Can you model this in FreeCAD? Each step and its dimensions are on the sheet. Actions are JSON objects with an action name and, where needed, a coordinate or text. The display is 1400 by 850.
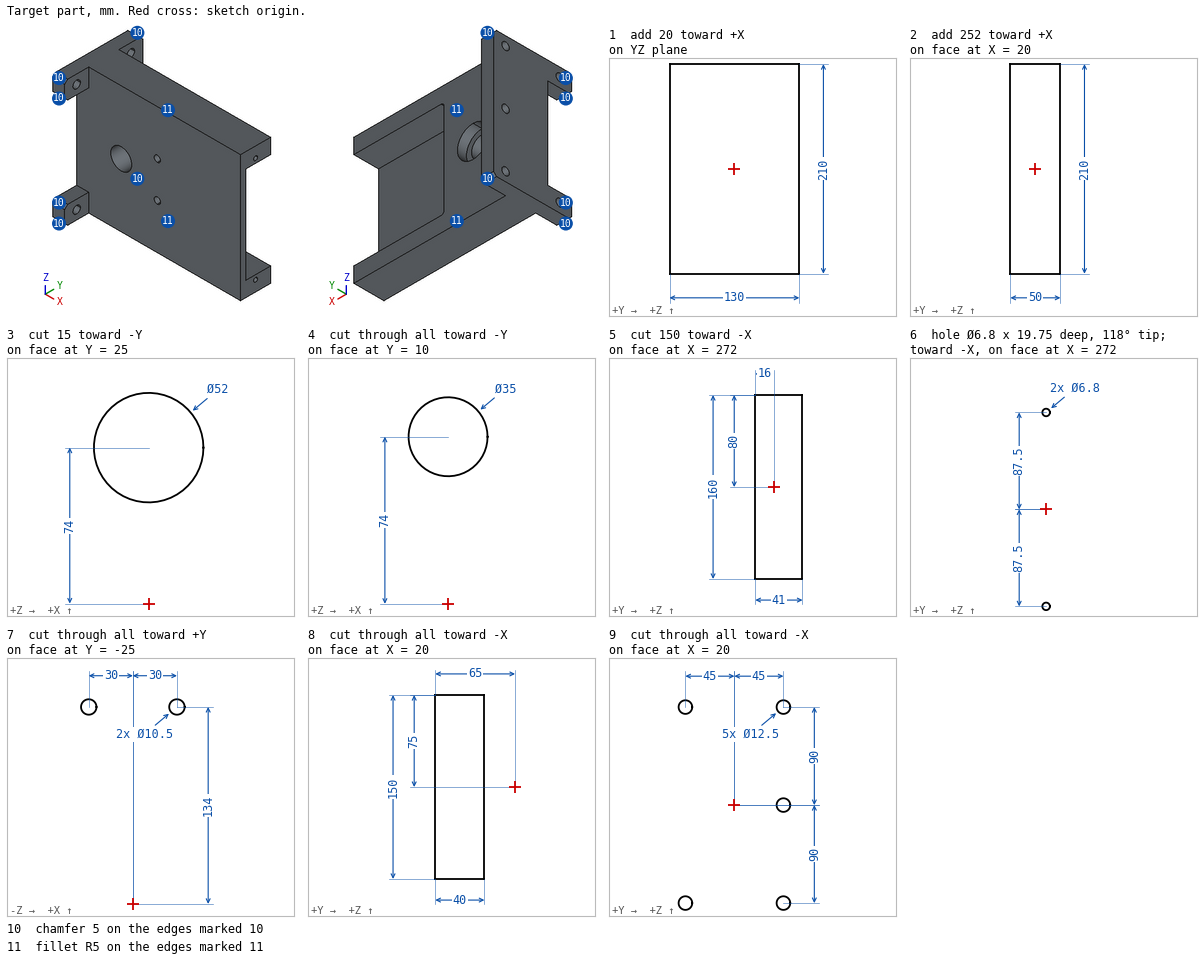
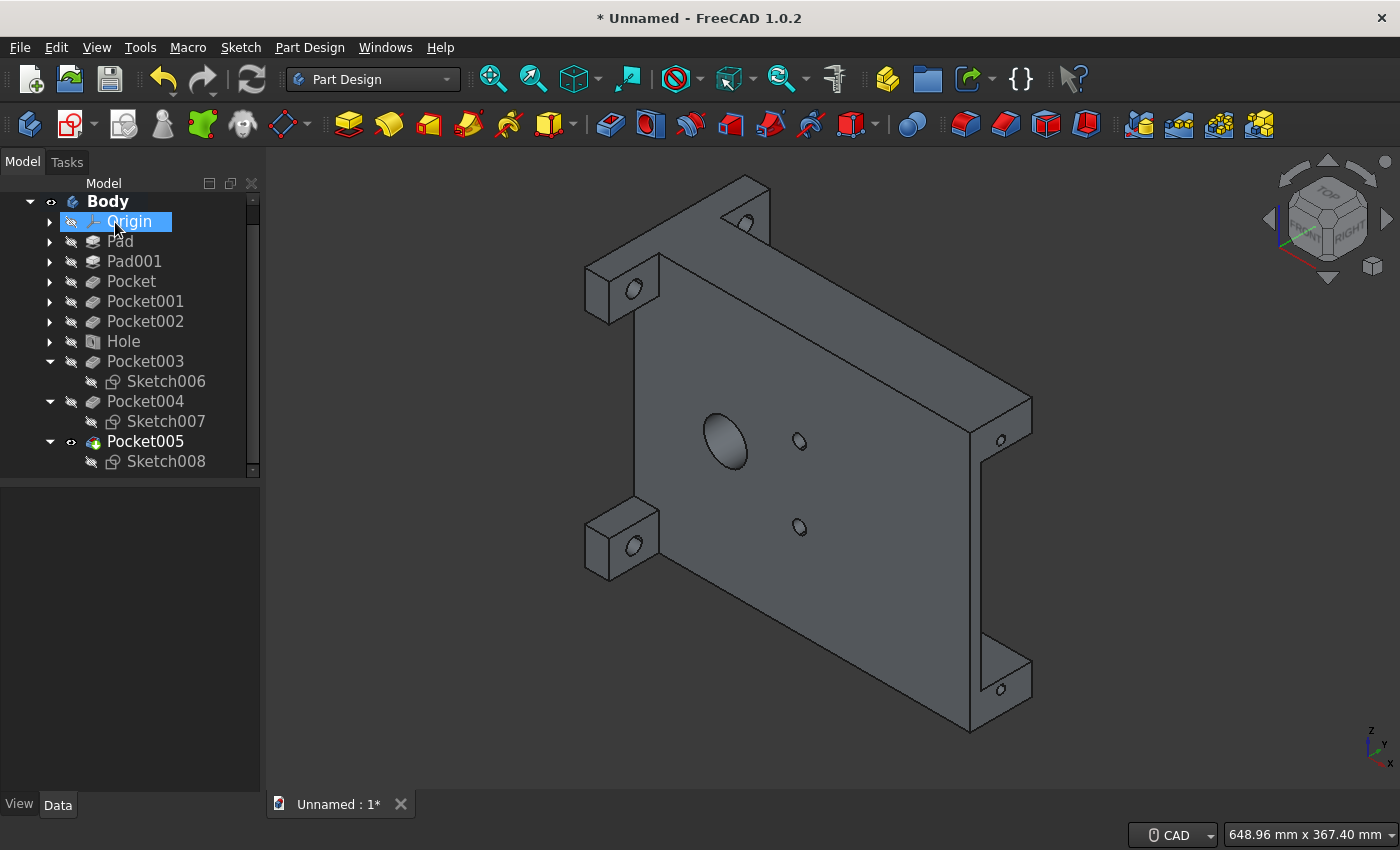
{"action": "left_click", "coordinate": [597, 274]}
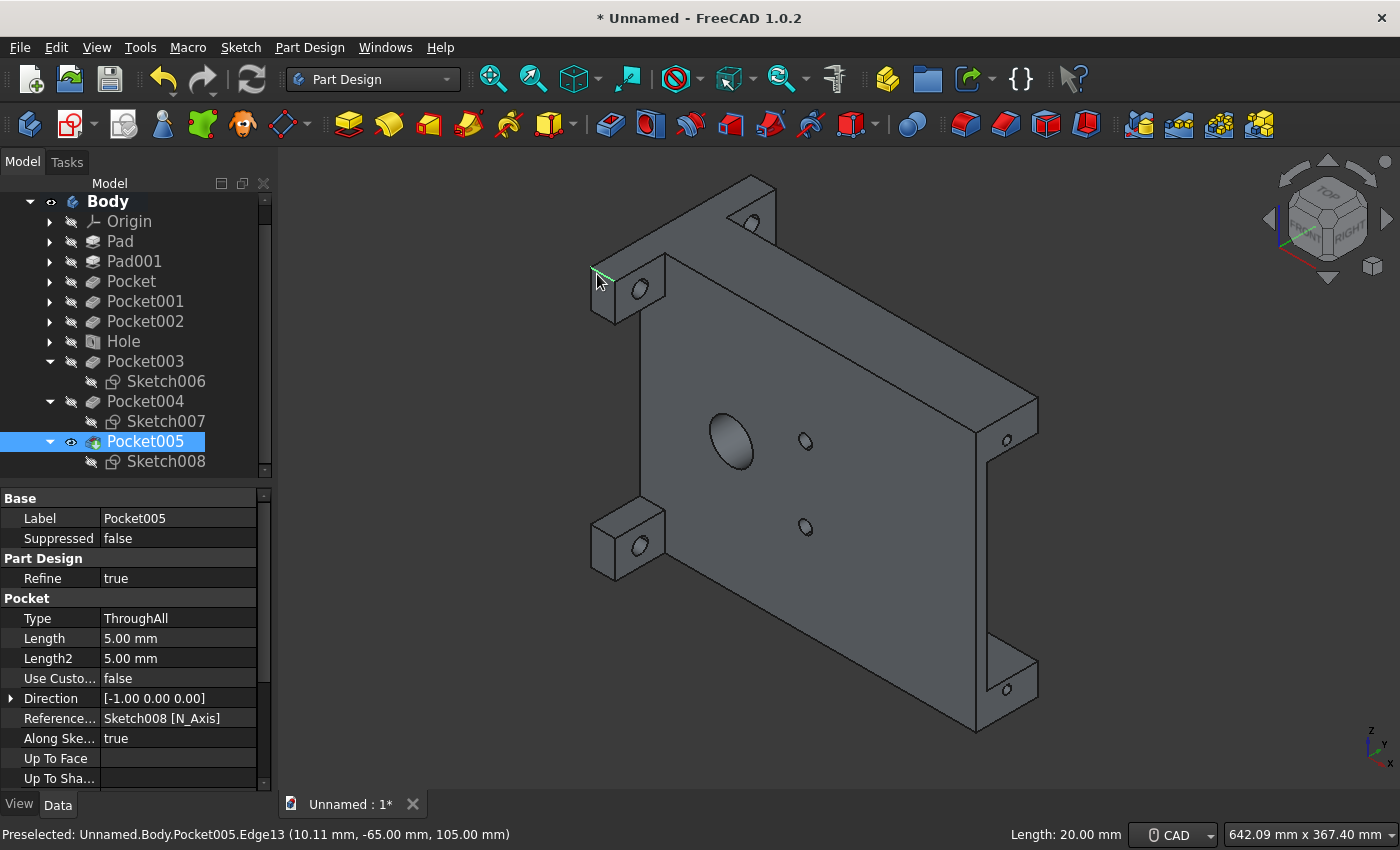
{"action": "left_click", "coordinate": [603, 530], "text": "ctrl"}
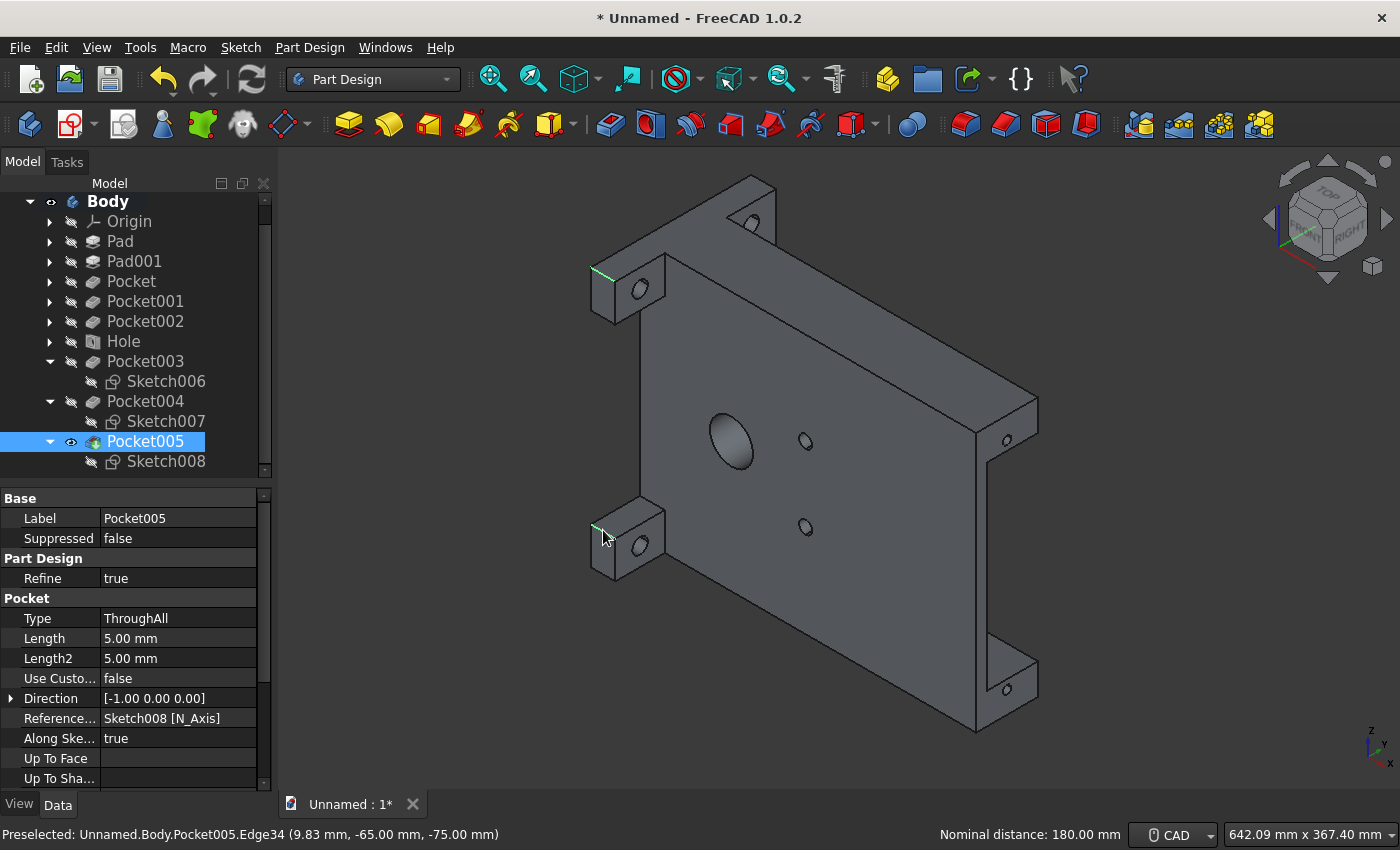
{"action": "key", "text": "2"}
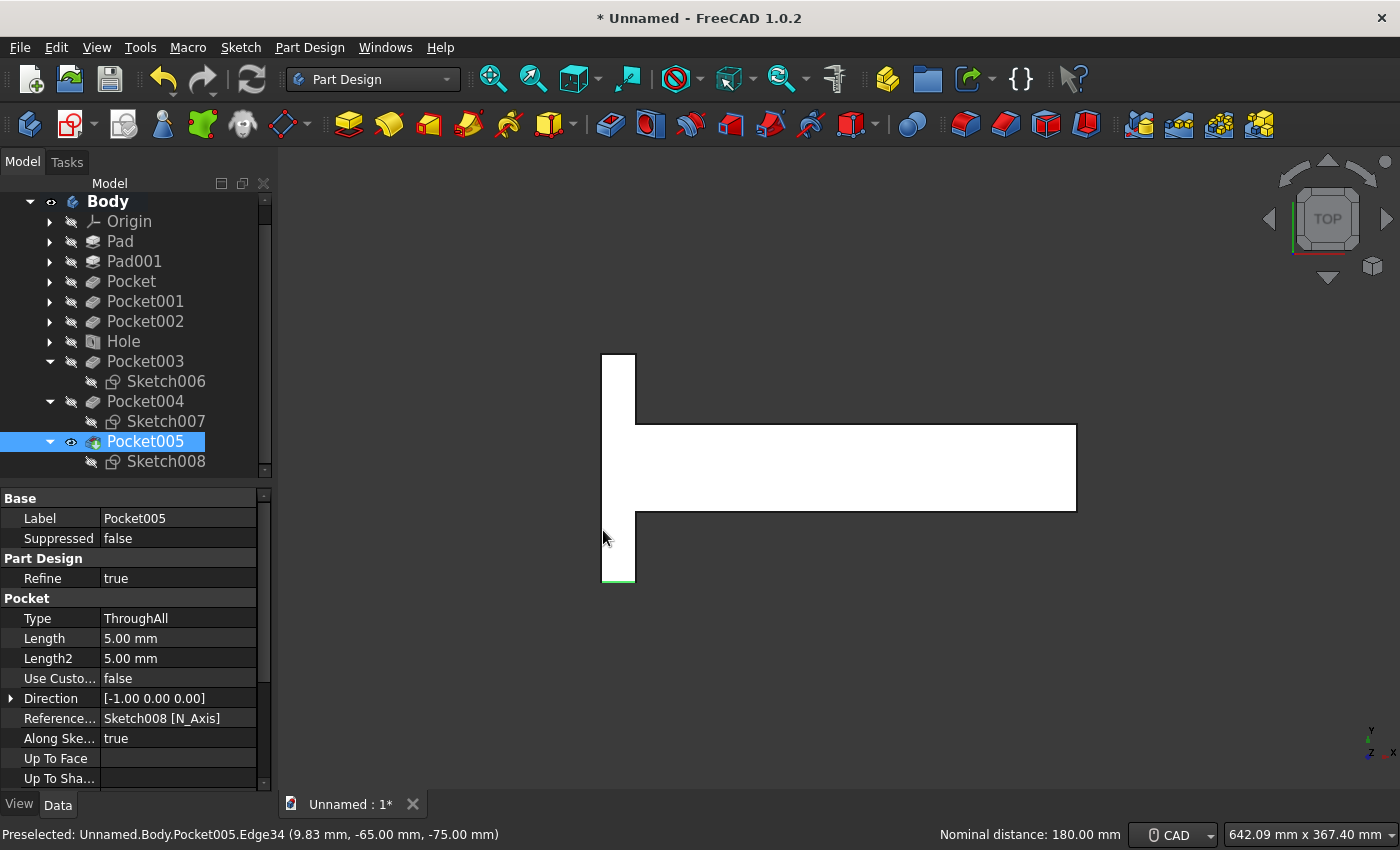
{"action": "left_click", "coordinate": [494, 80]}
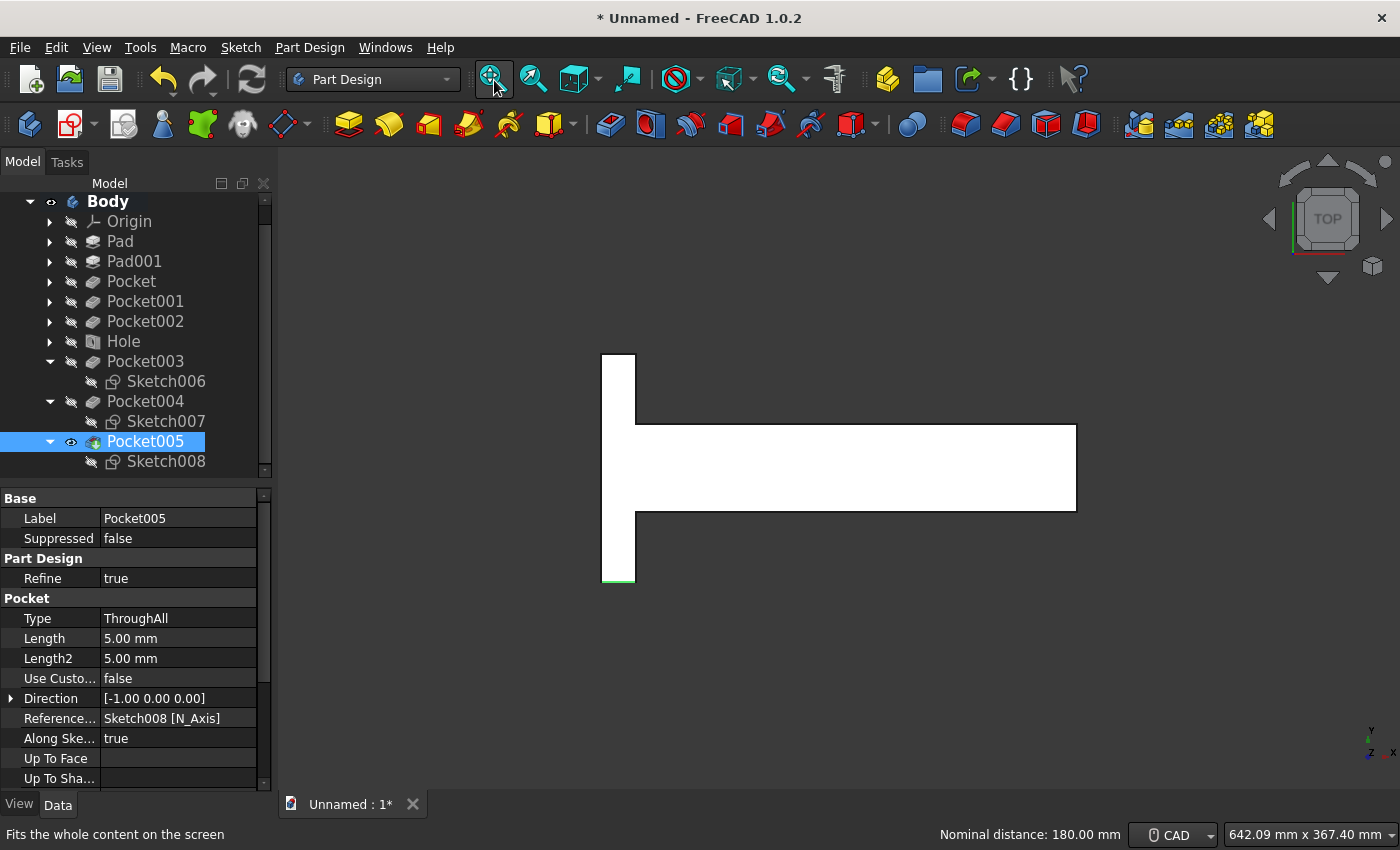
{"action": "left_click", "coordinate": [619, 353], "text": "ctrl"}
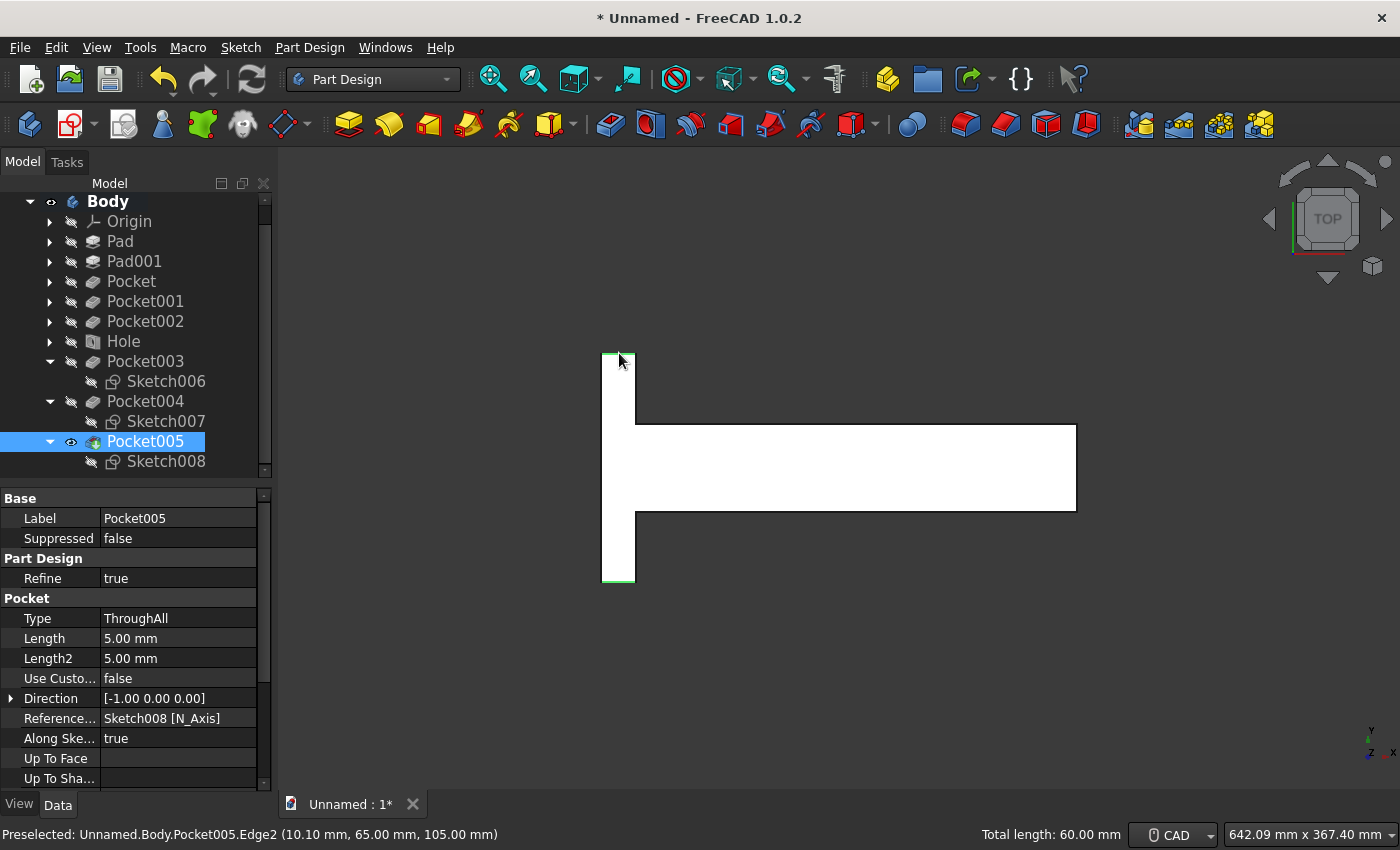
{"action": "key", "text": "1"}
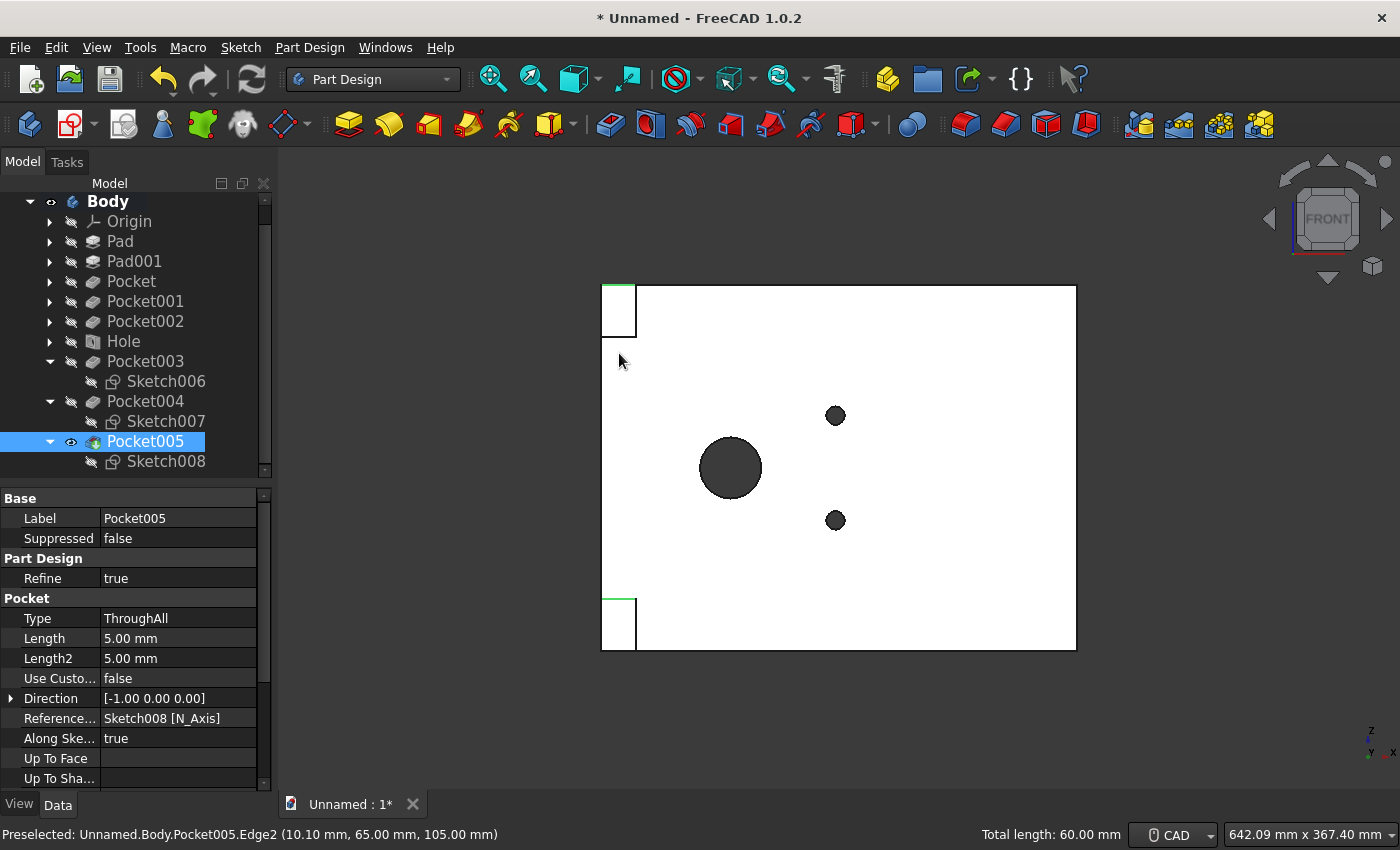
{"action": "left_click", "coordinate": [619, 650], "text": "ctrl"}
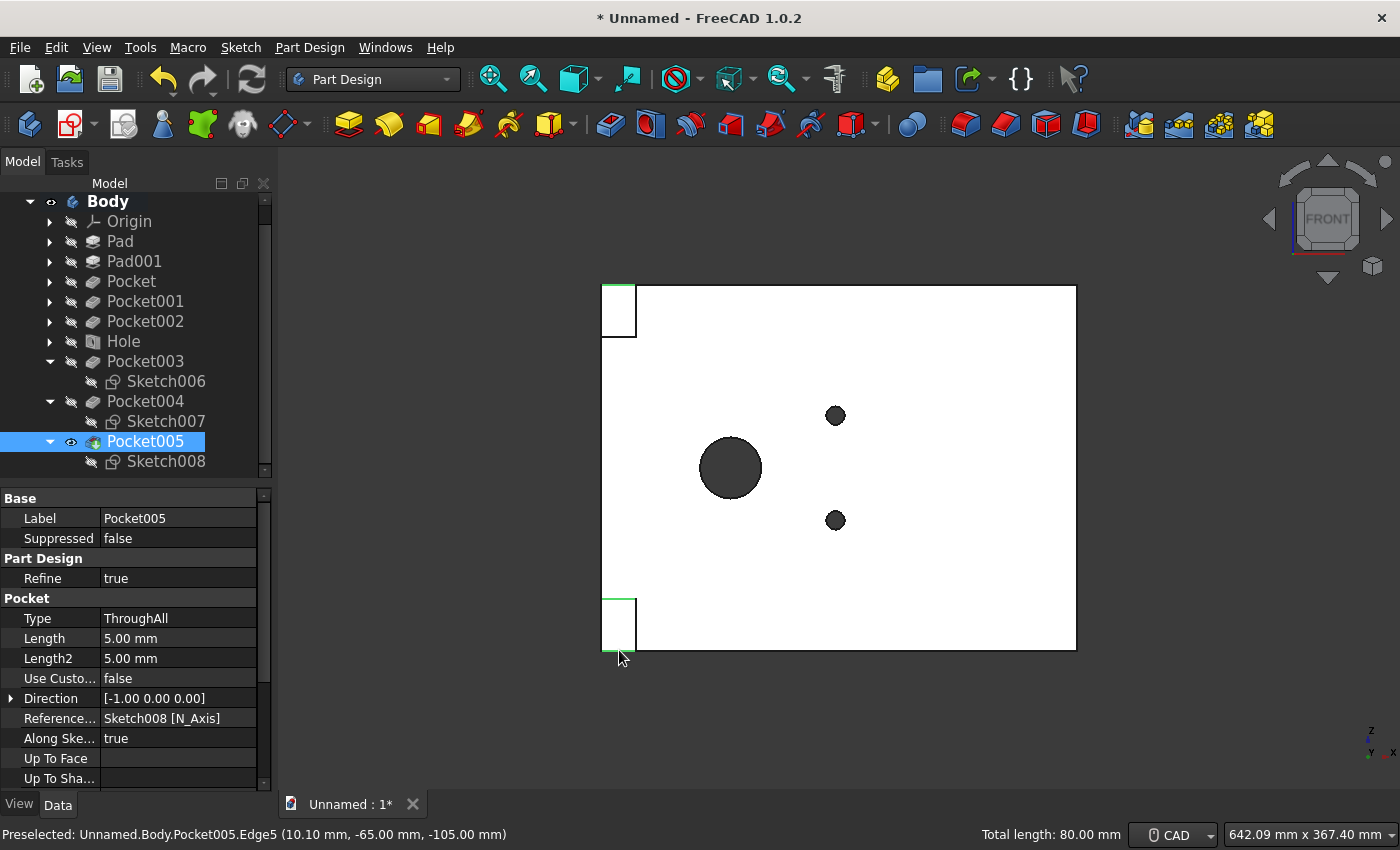
{"action": "left_click", "coordinate": [619, 336], "text": "ctrl"}